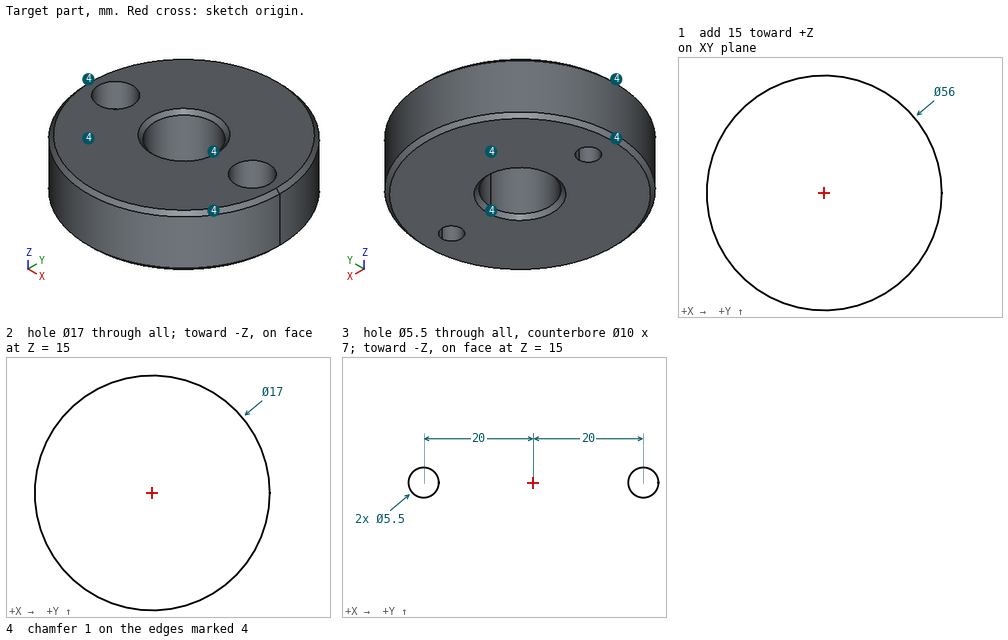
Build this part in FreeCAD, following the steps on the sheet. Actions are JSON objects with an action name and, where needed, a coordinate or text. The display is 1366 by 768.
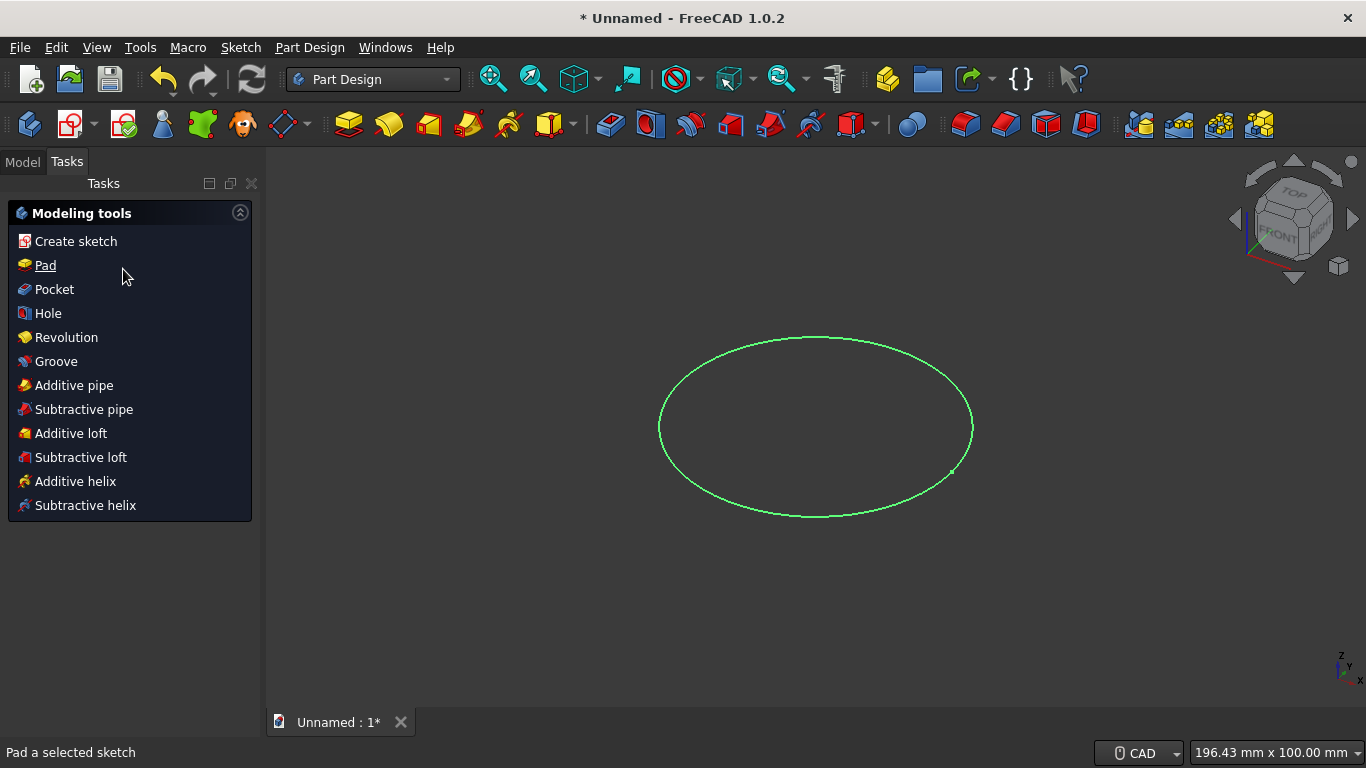
{"action": "left_click", "coordinate": [350, 124]}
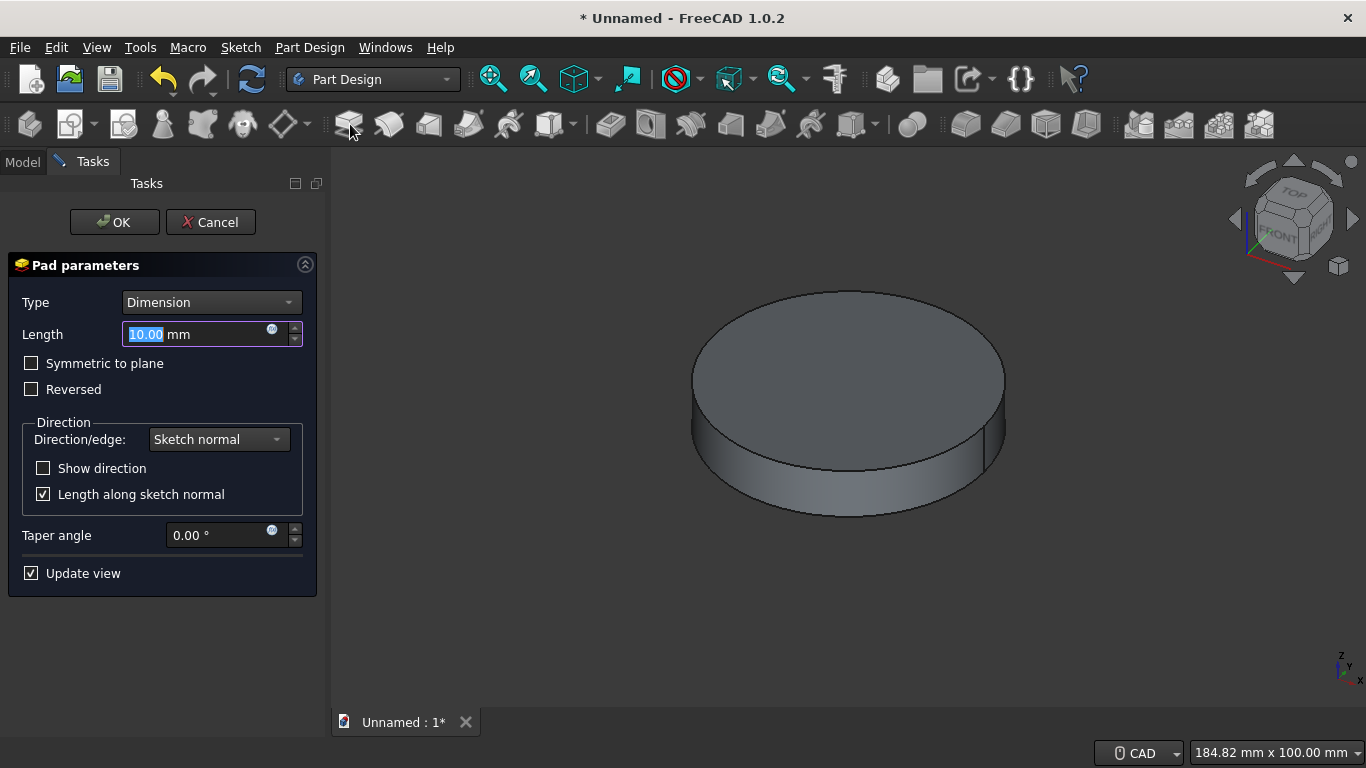
{"action": "type", "text": "15"}
{"action": "key", "text": "Tab"}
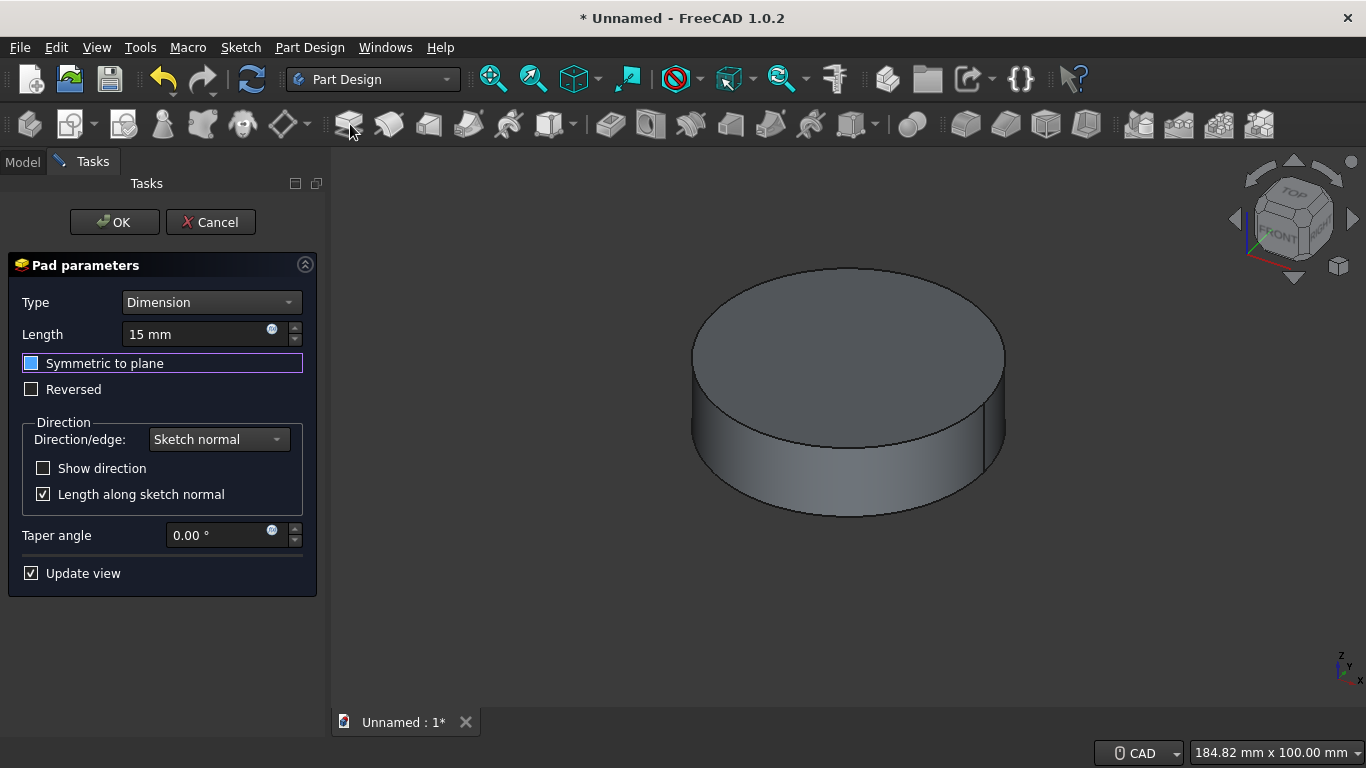
{"action": "left_click", "coordinate": [115, 222]}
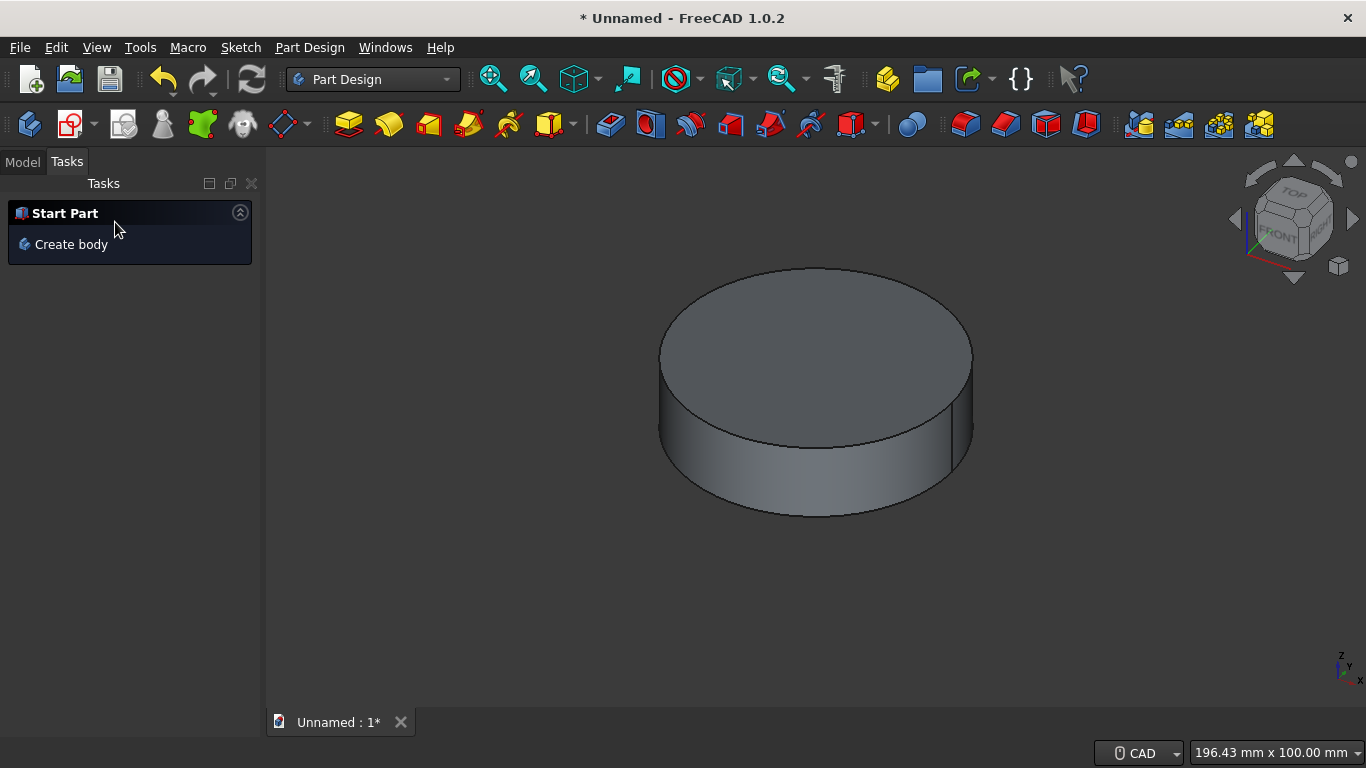
{"action": "left_click", "coordinate": [816, 357]}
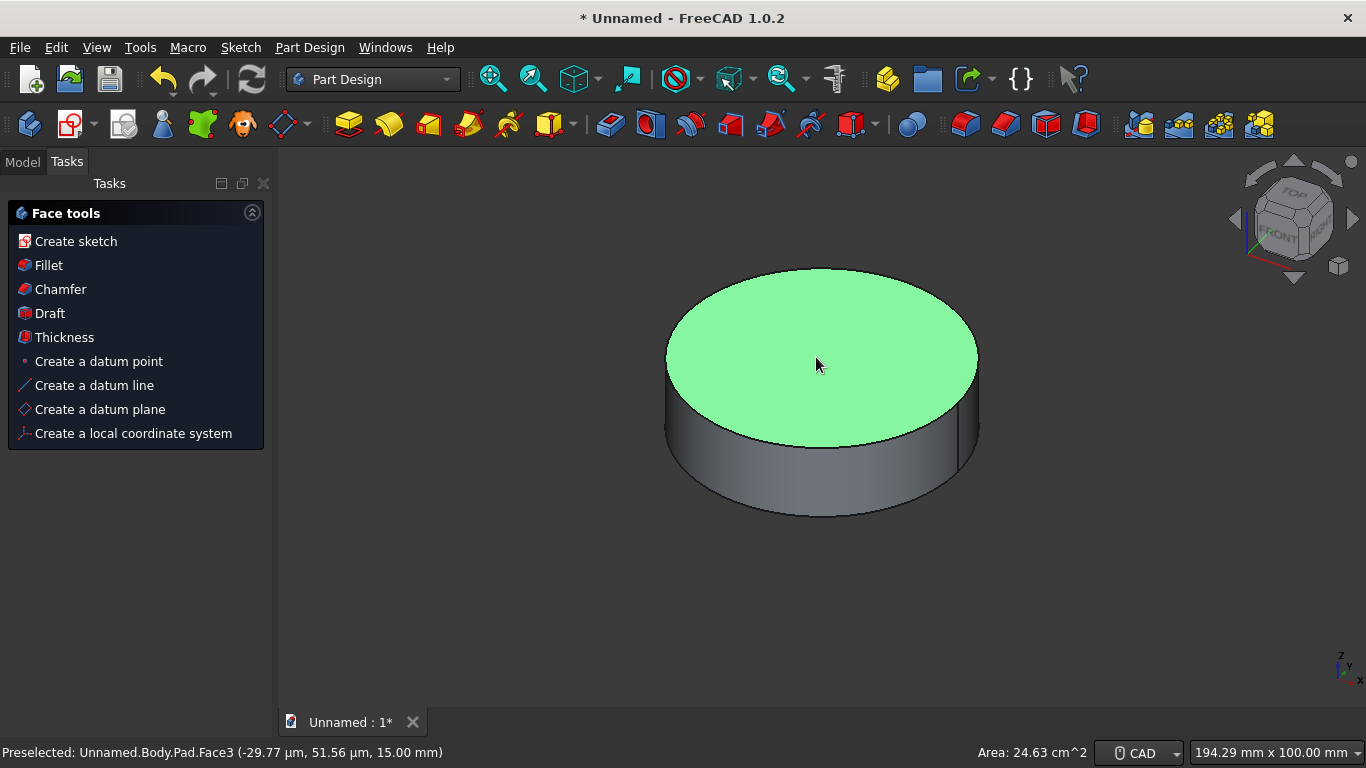
{"action": "left_click", "coordinate": [70, 124]}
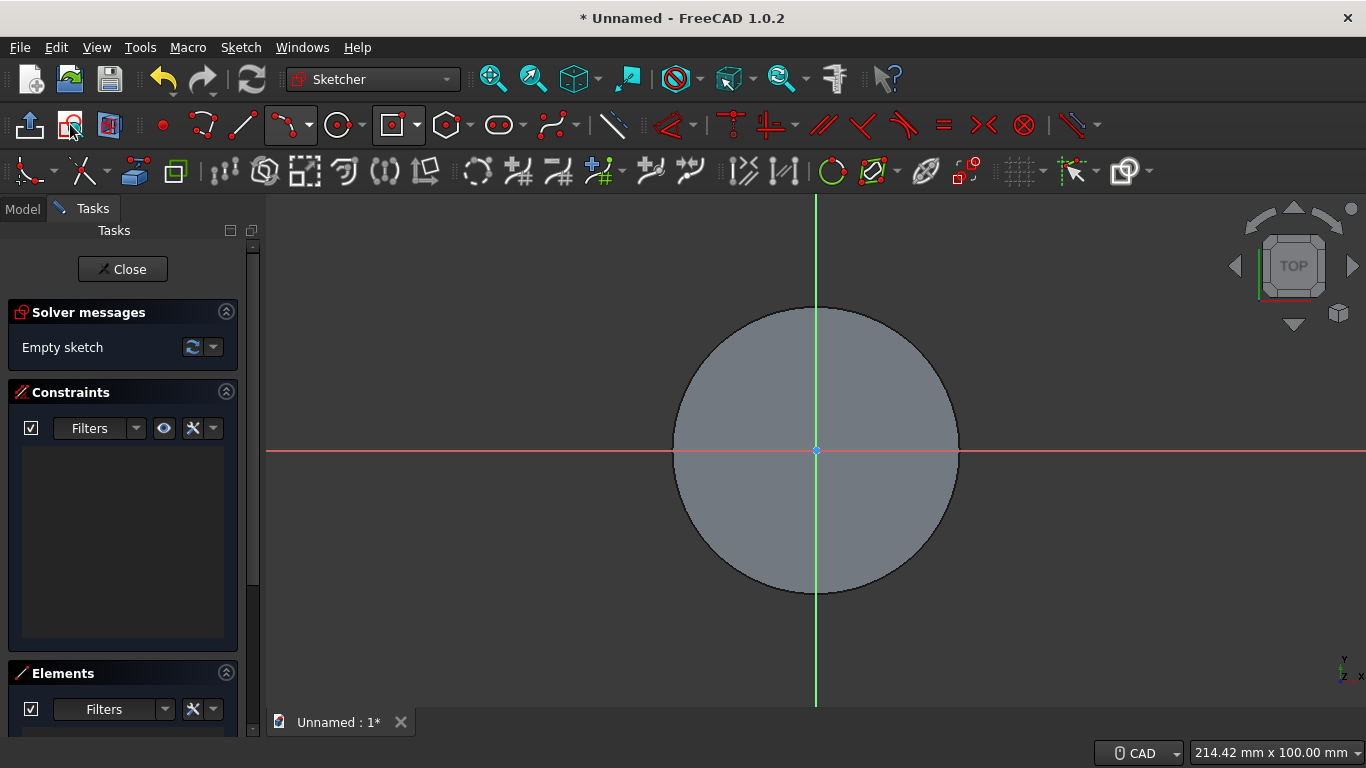
{"action": "scroll", "coordinate": [838, 450], "scroll_direction": "up", "scroll_amount": 7}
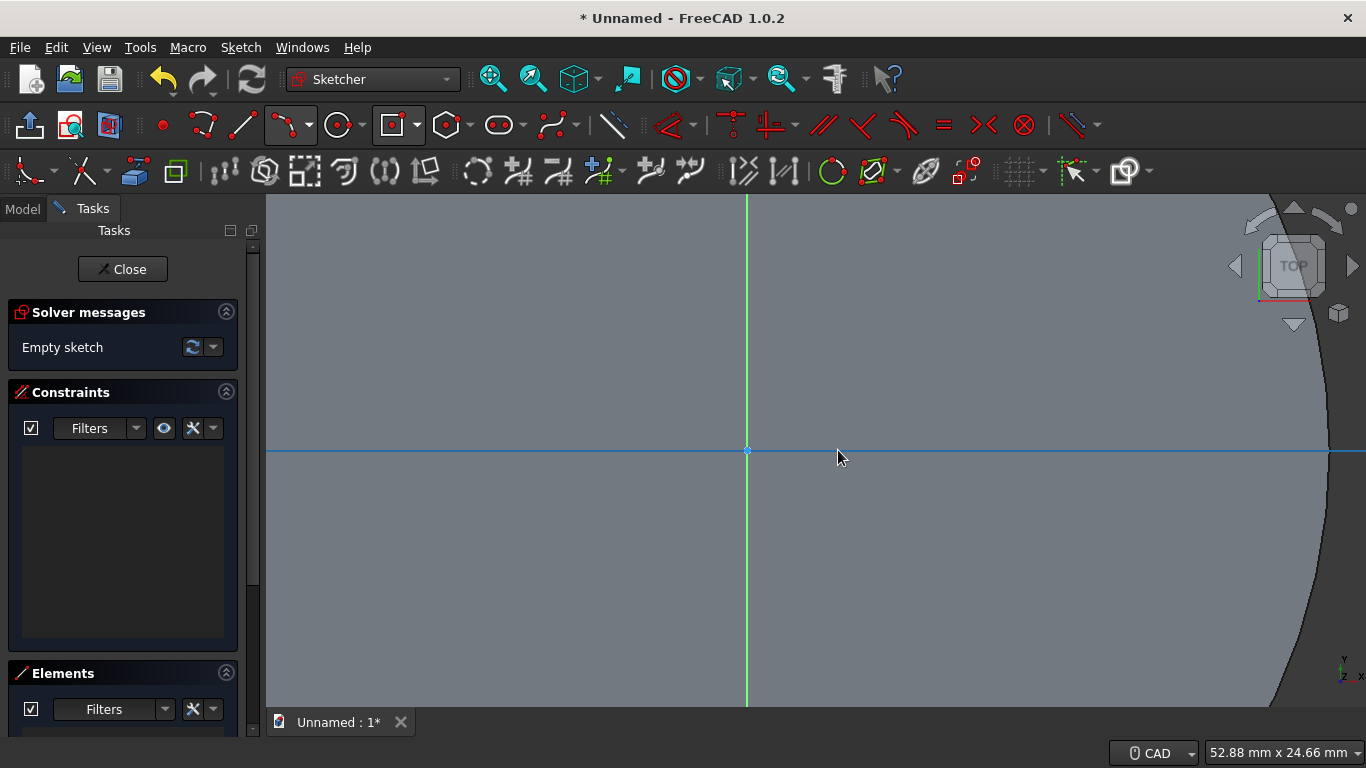
{"action": "left_click", "coordinate": [338, 126]}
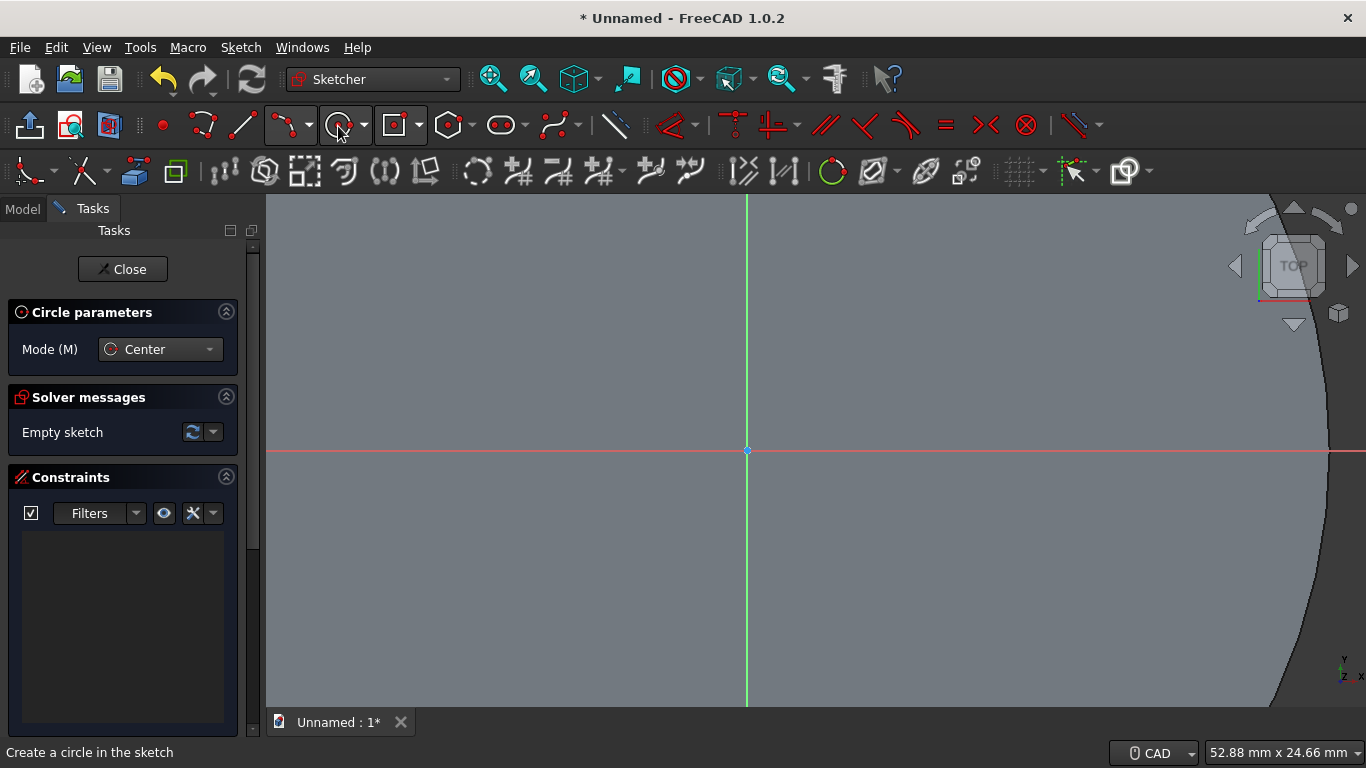
{"action": "left_click", "coordinate": [747, 450]}
{"action": "left_click", "coordinate": [872, 325]}
{"action": "key", "text": "Escape"}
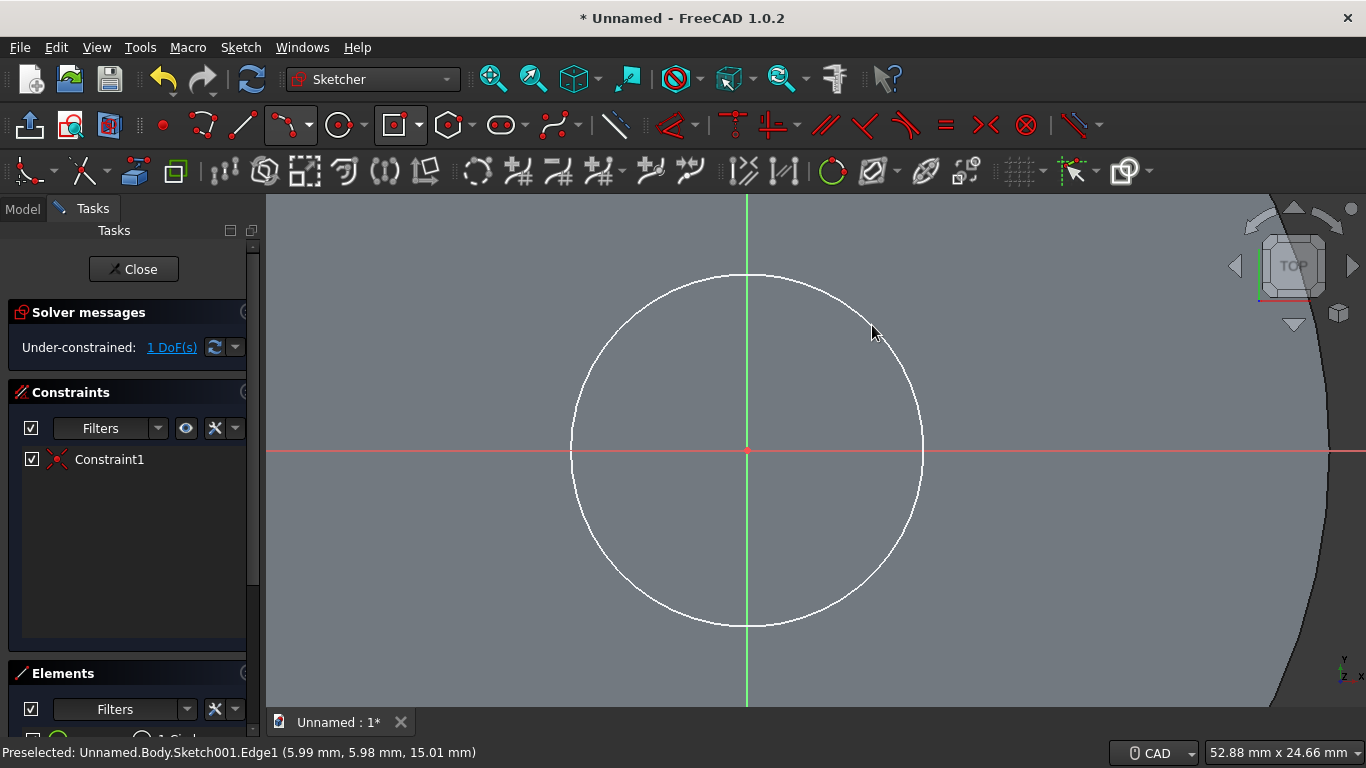
{"action": "left_click", "coordinate": [670, 126]}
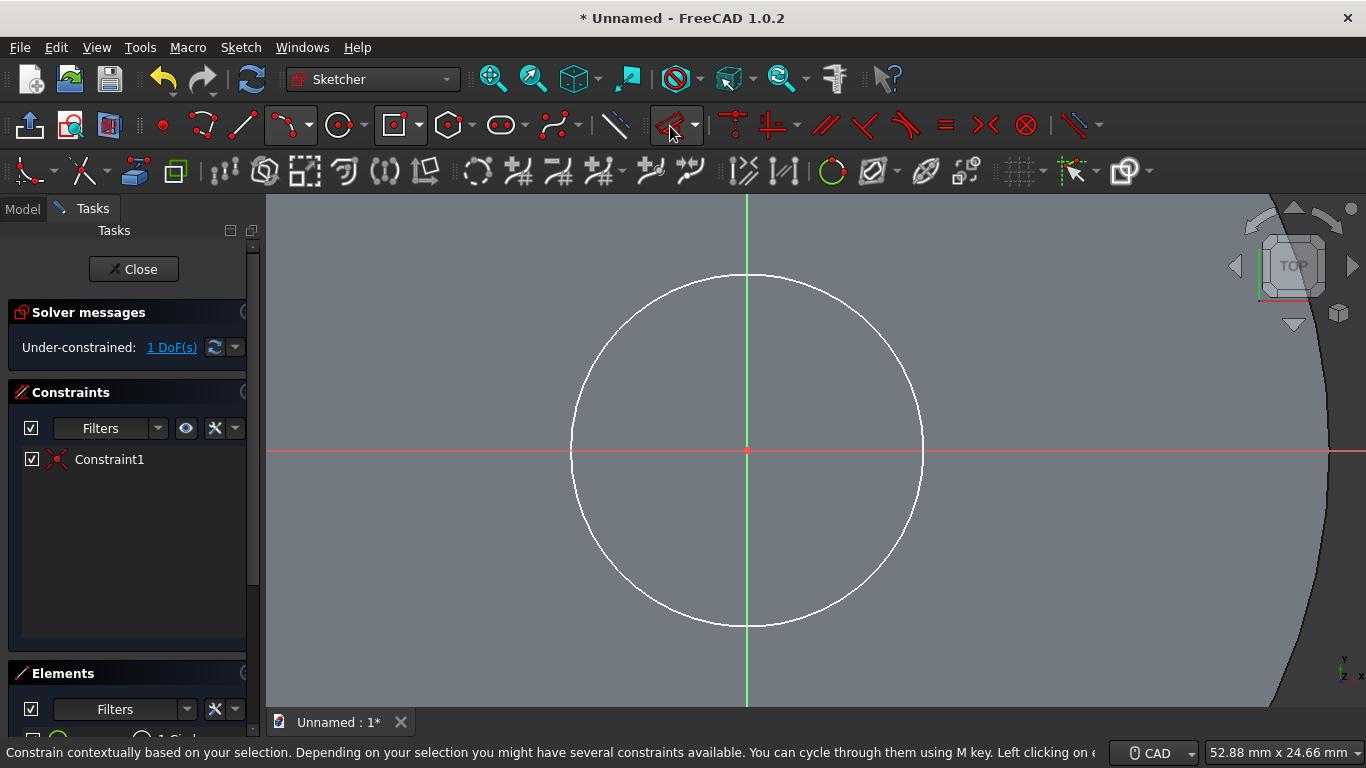
{"action": "left_click", "coordinate": [871, 325]}
{"action": "left_click", "coordinate": [893, 302]}